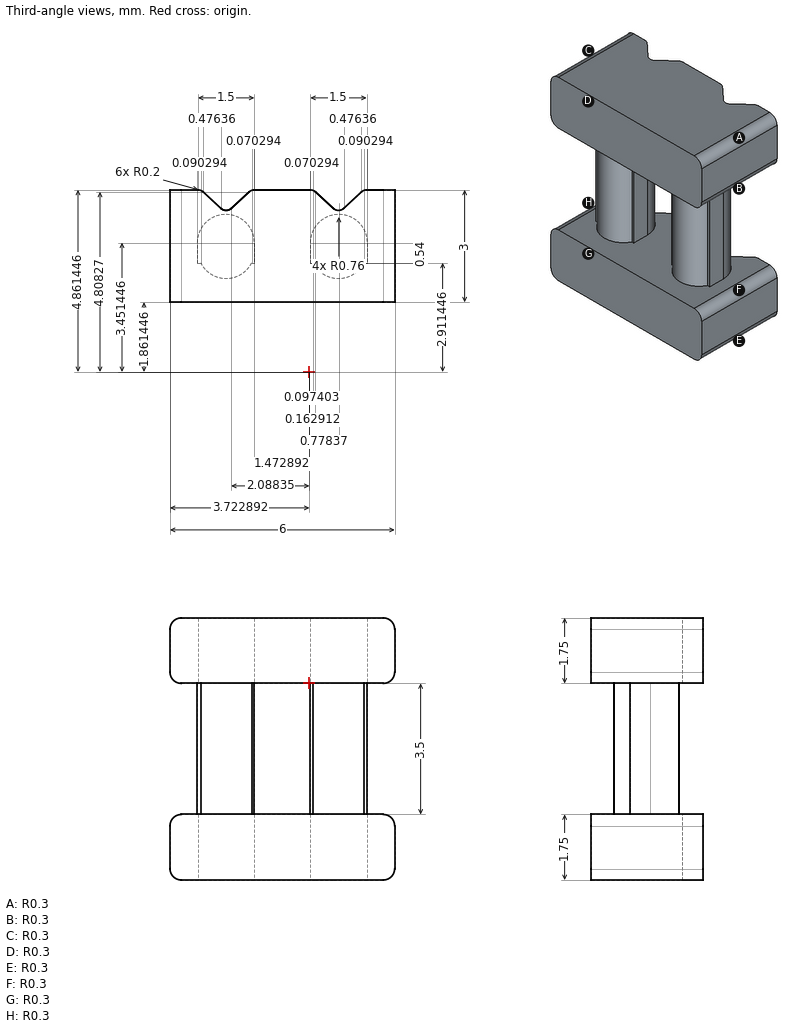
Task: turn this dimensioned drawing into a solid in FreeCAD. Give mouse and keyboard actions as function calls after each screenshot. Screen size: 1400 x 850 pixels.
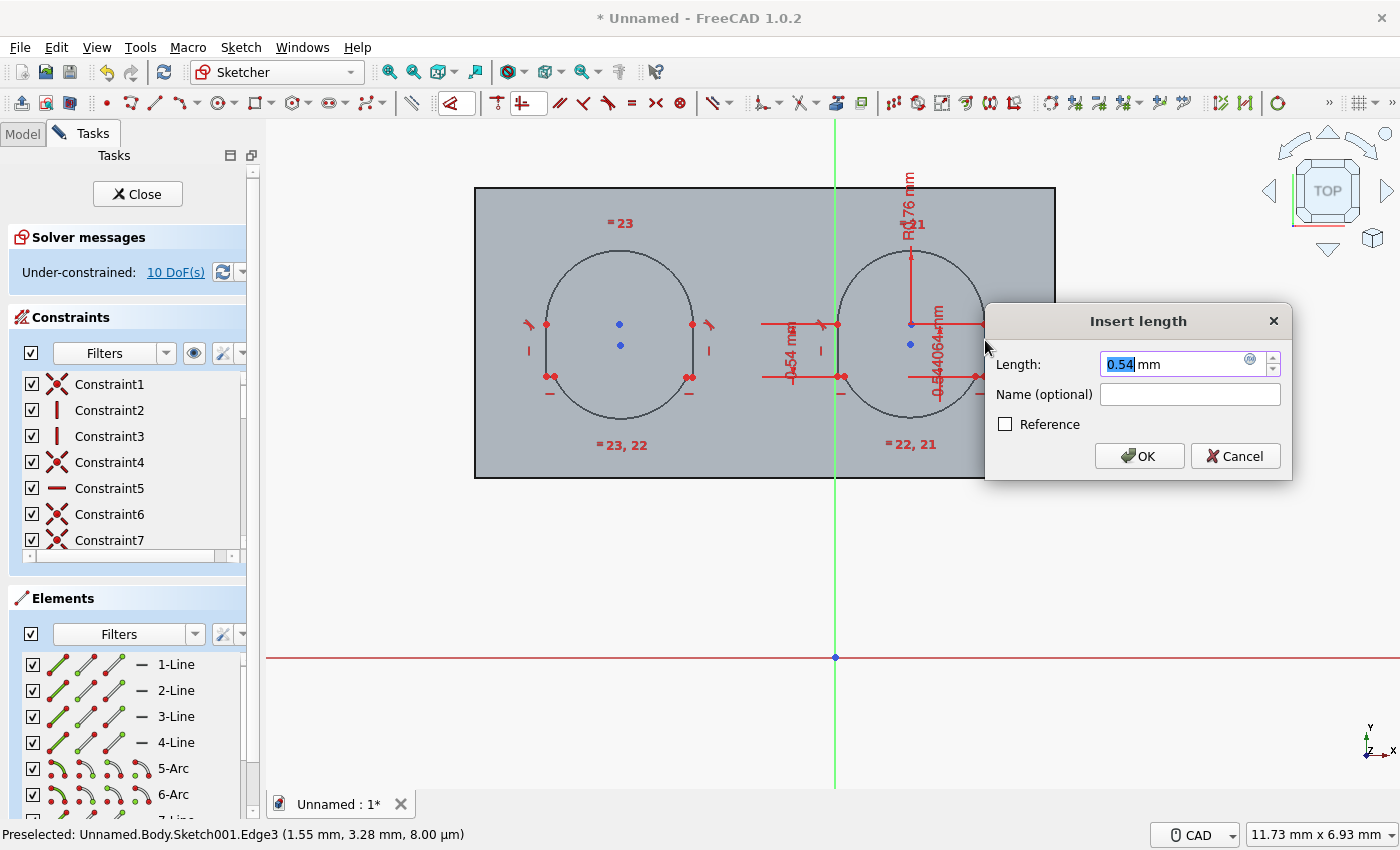
text(0.54)
key(Return)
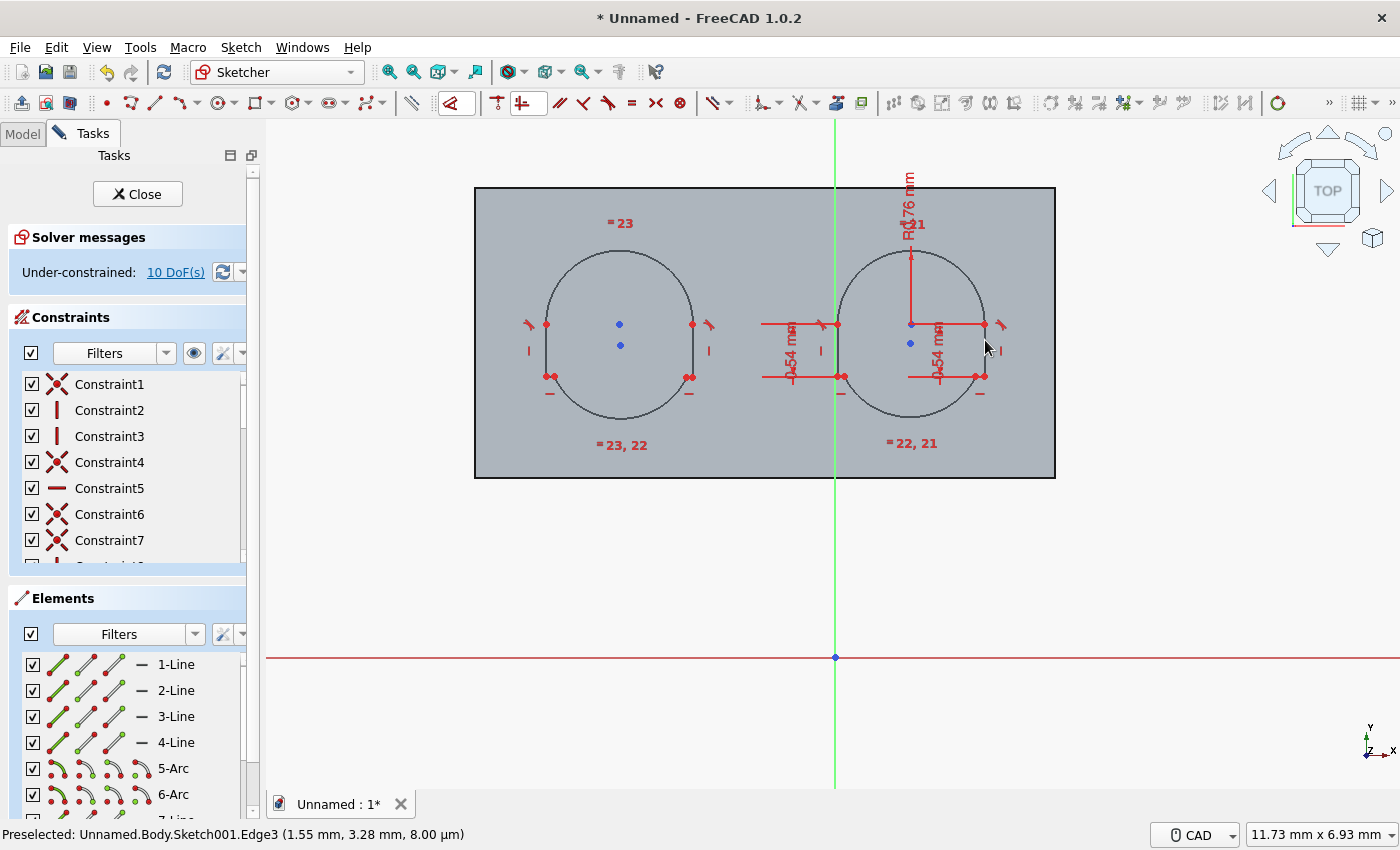
click(693, 340)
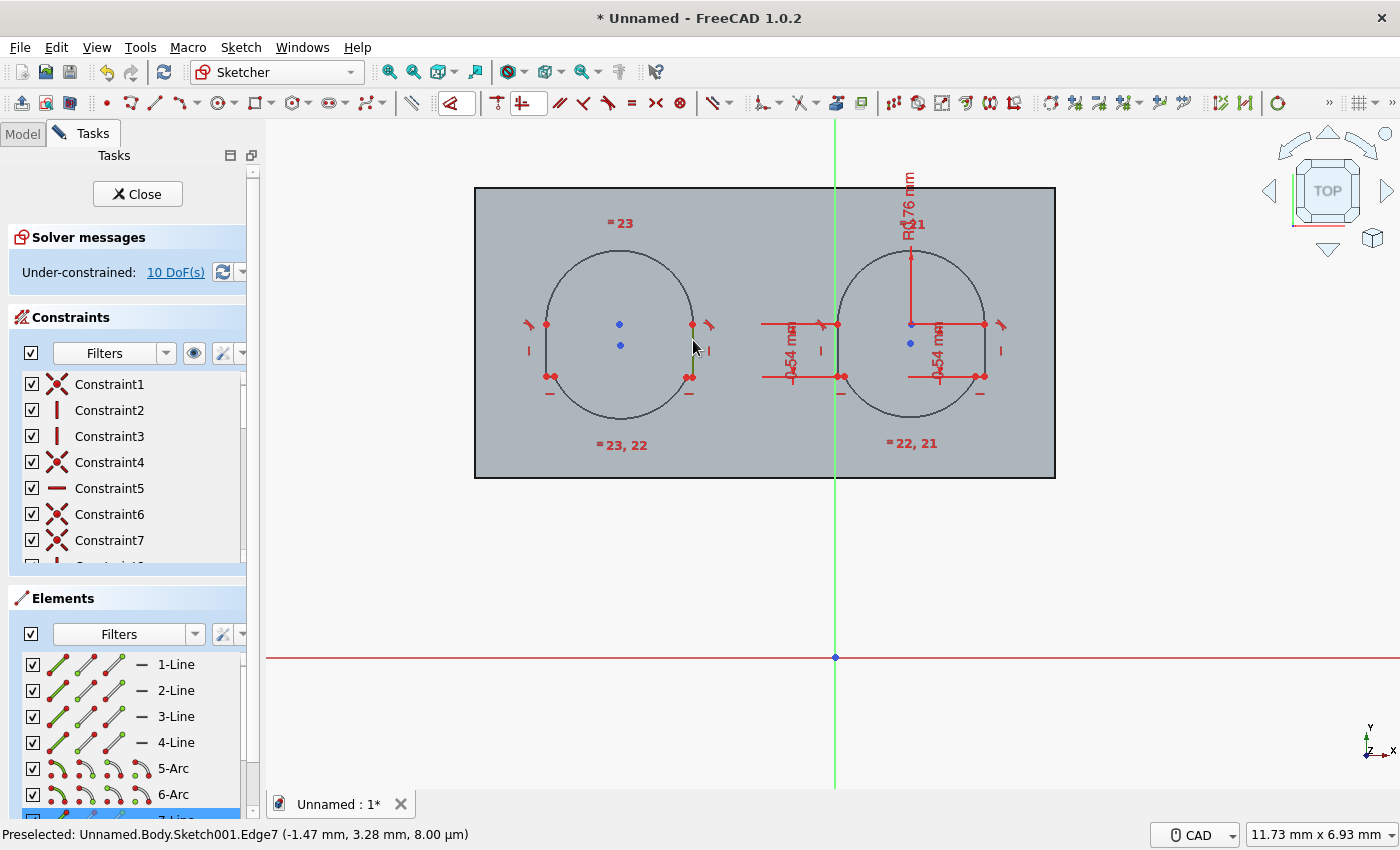
click(470, 104)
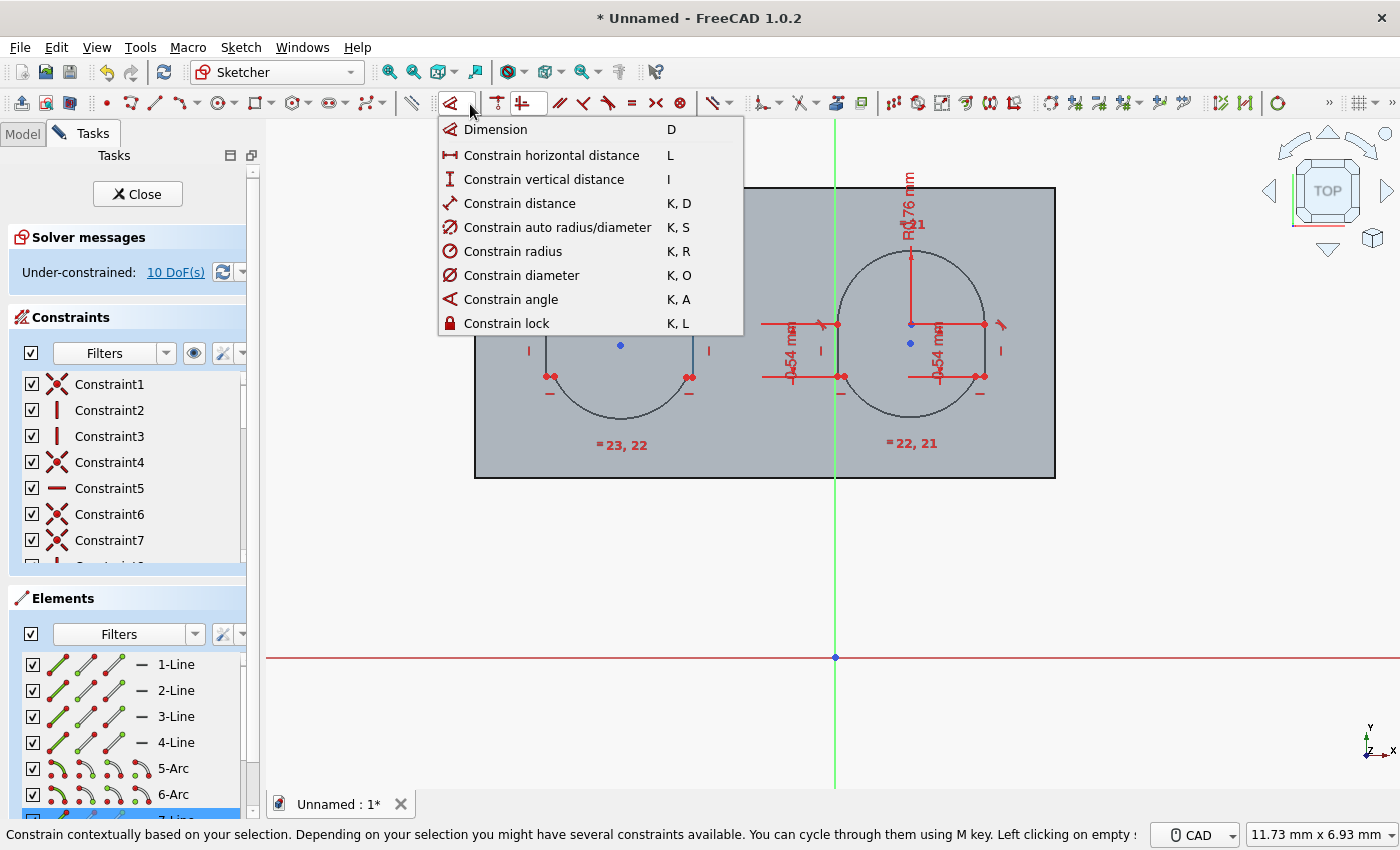
click(591, 179)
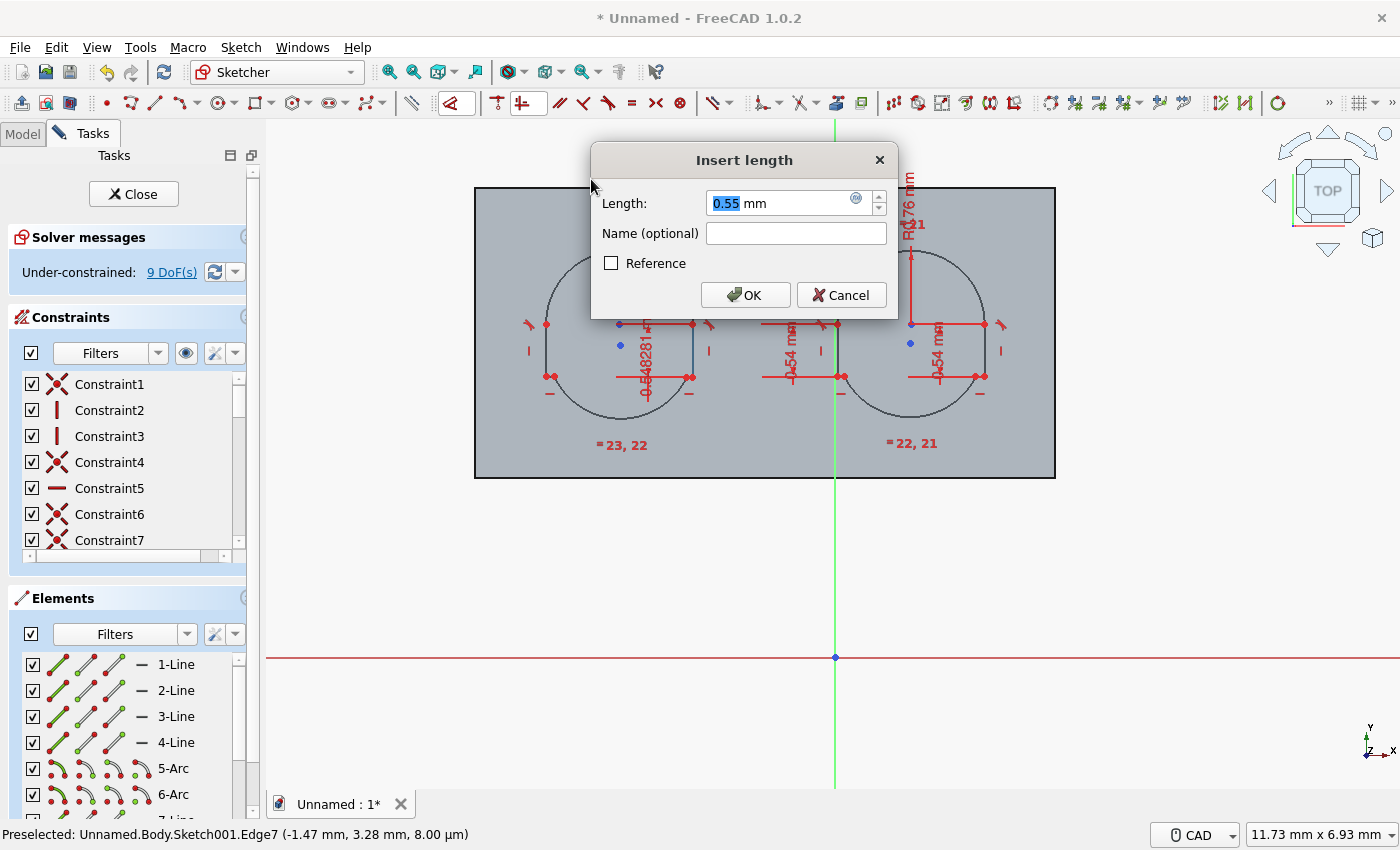
text(0.54)
key(Return)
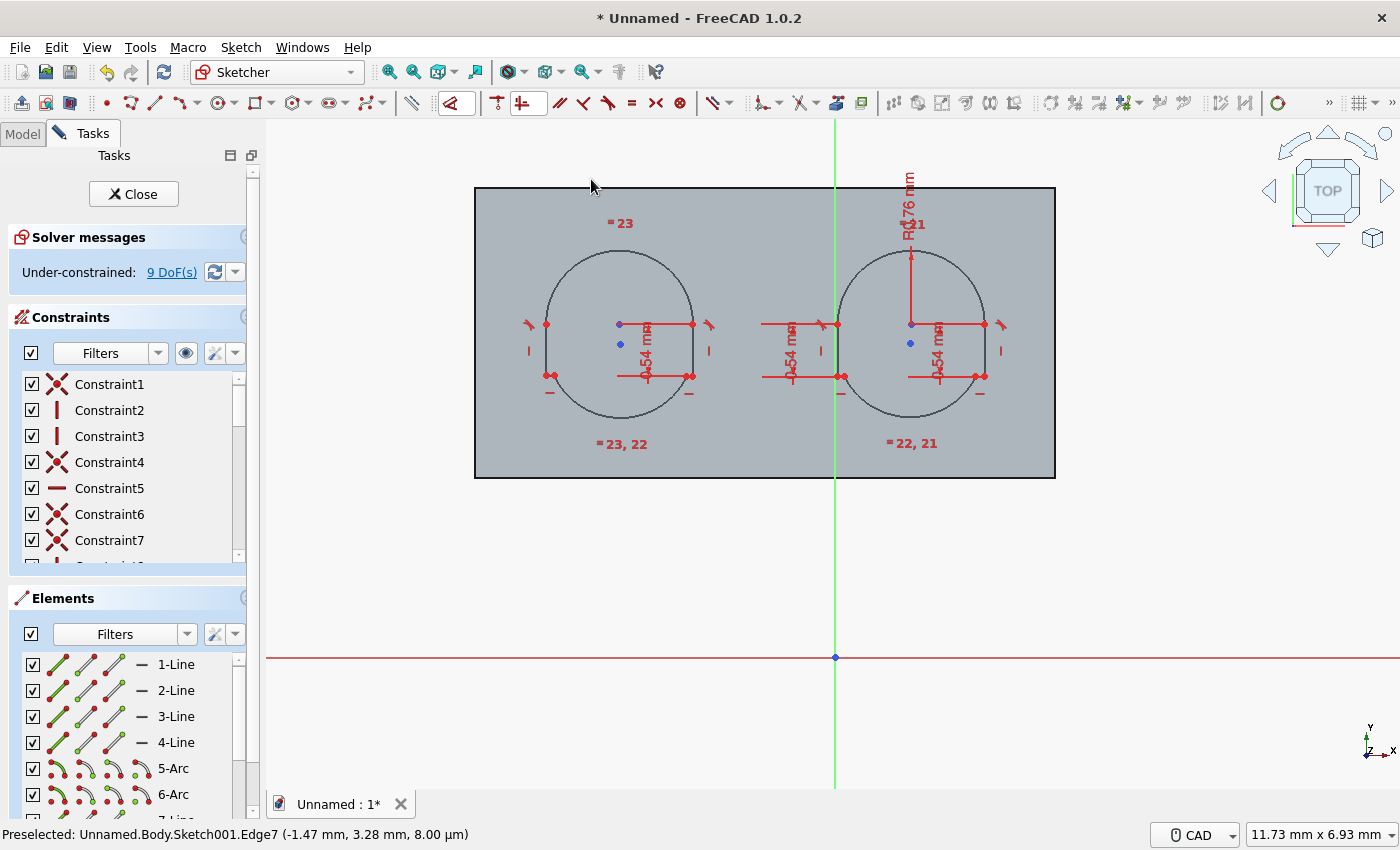
click(546, 360)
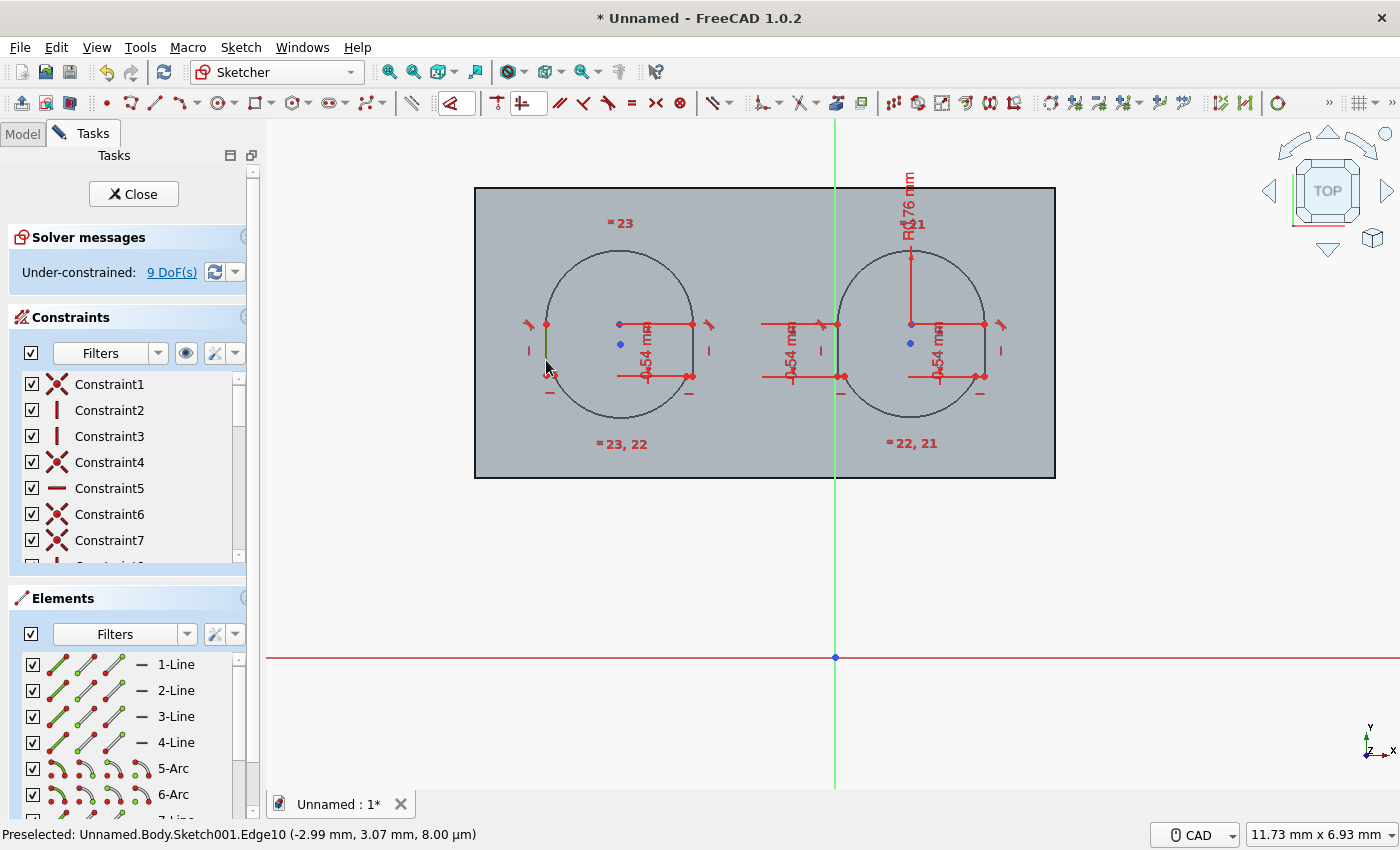
click(470, 104)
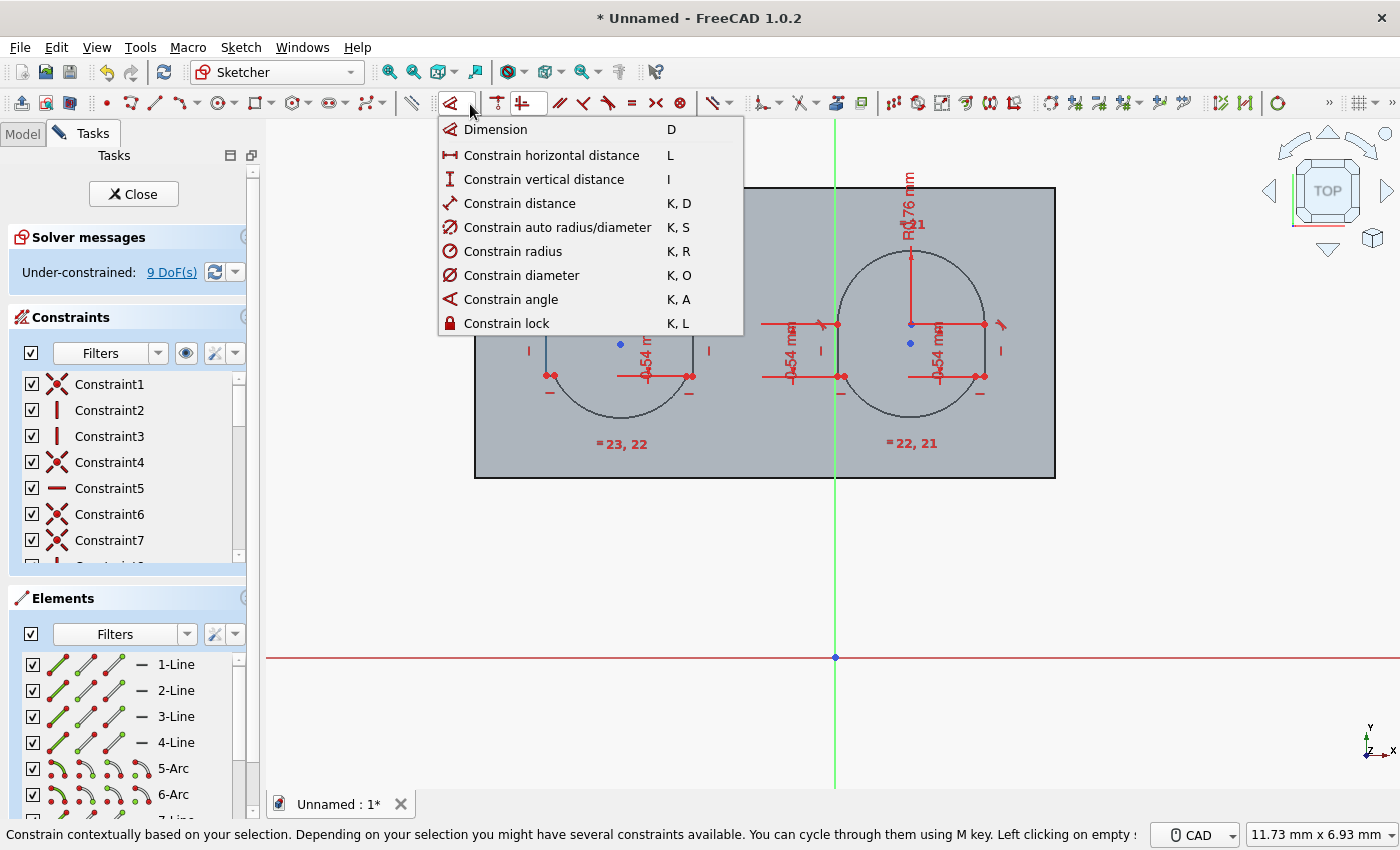
click(591, 179)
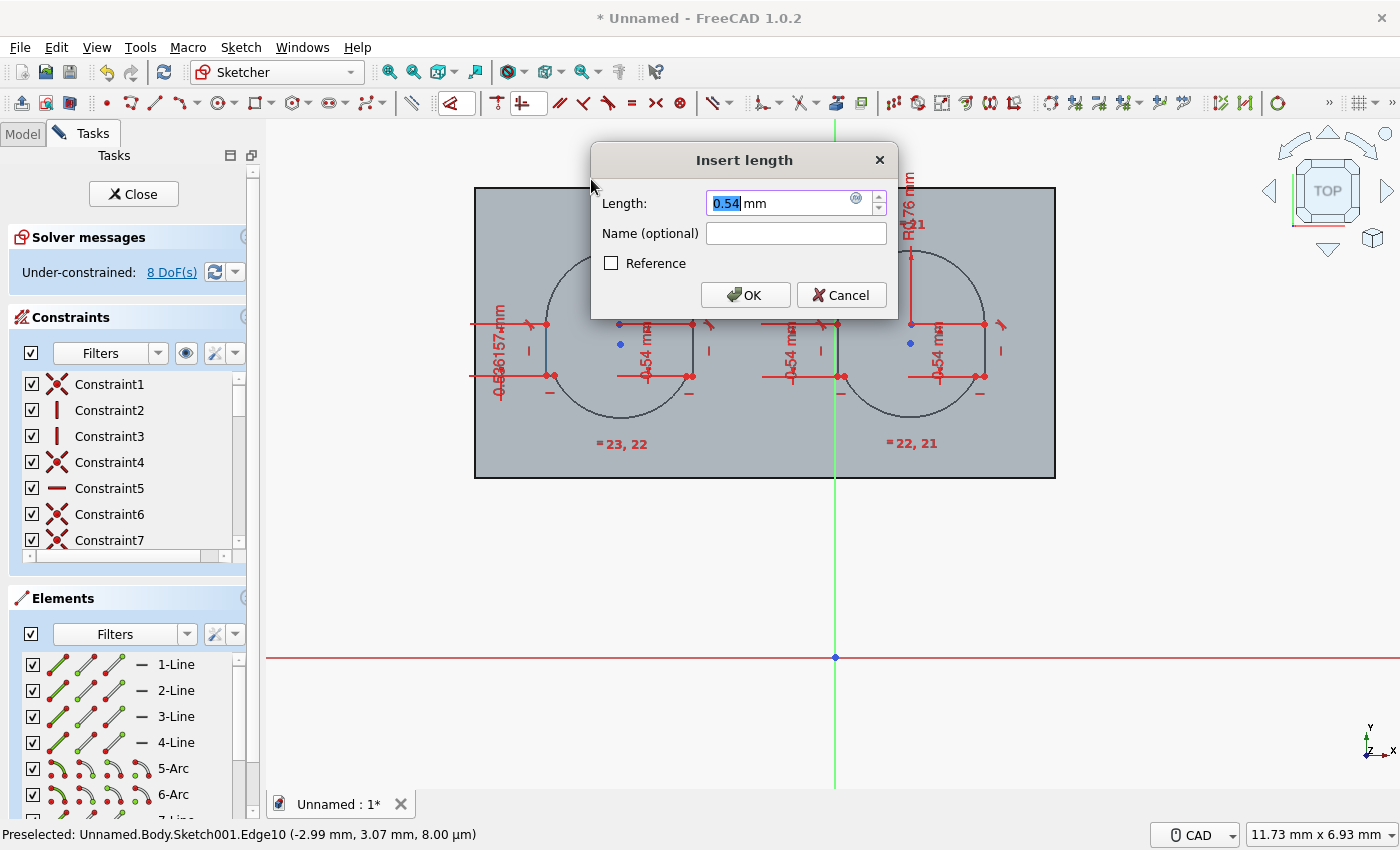
text(0.54)
key(Return)